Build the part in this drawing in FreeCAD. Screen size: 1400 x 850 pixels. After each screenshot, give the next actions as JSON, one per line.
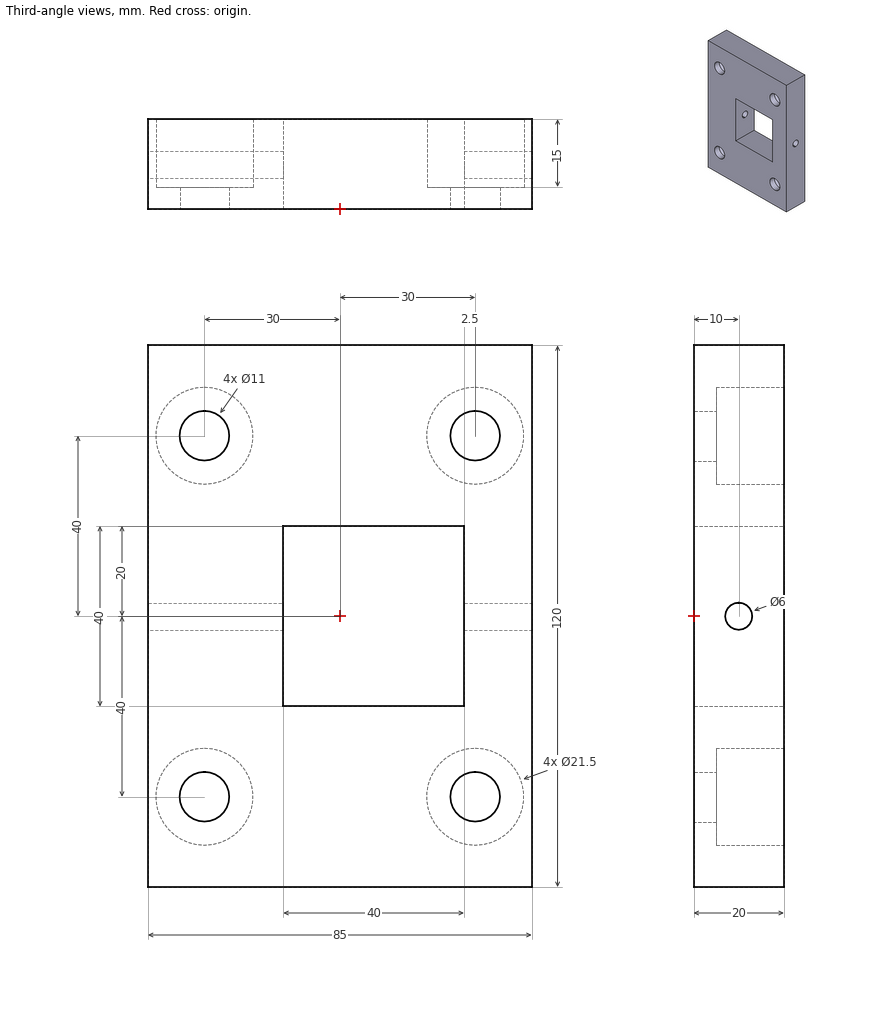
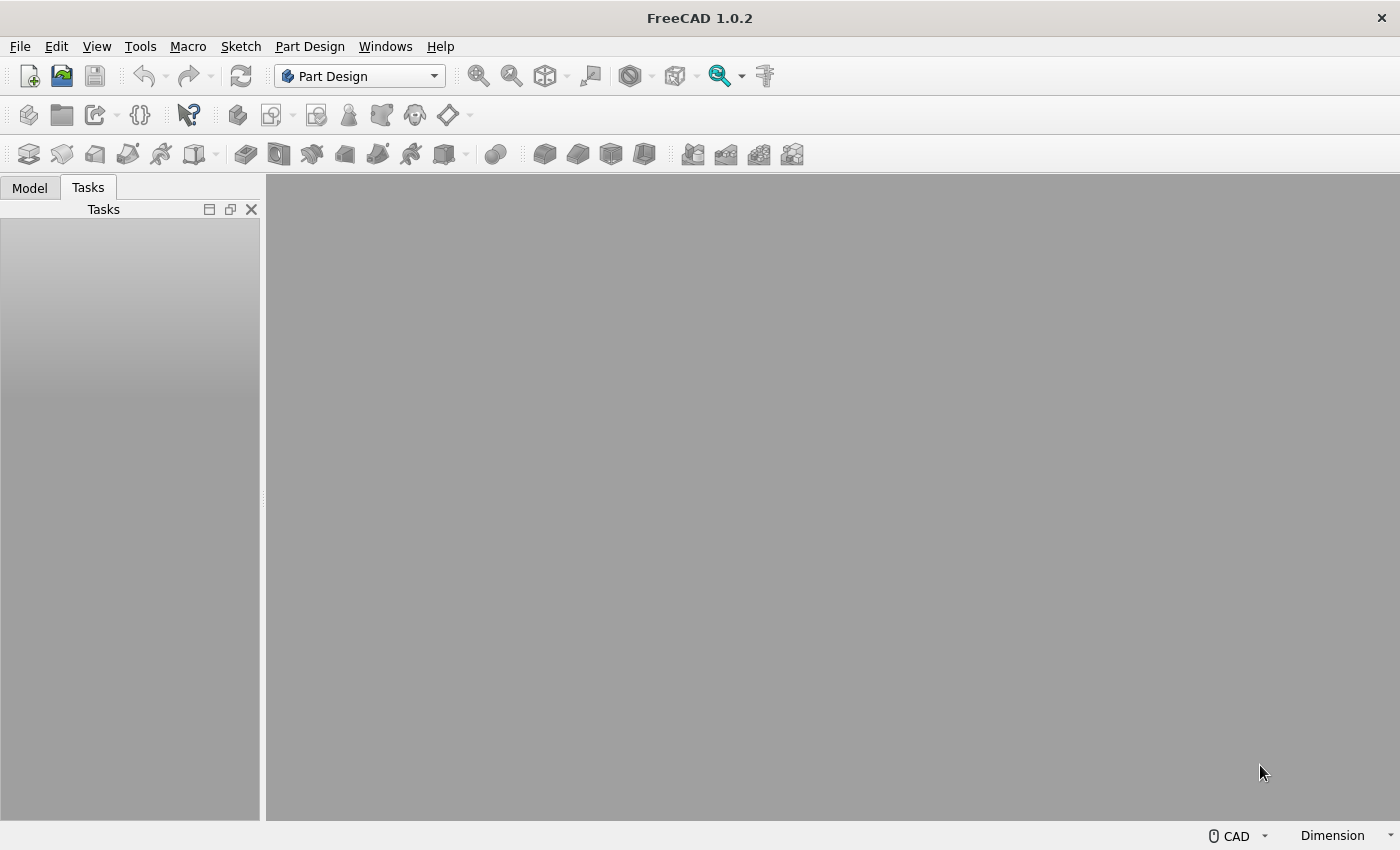
{"action": "key", "text": "ctrl+n"}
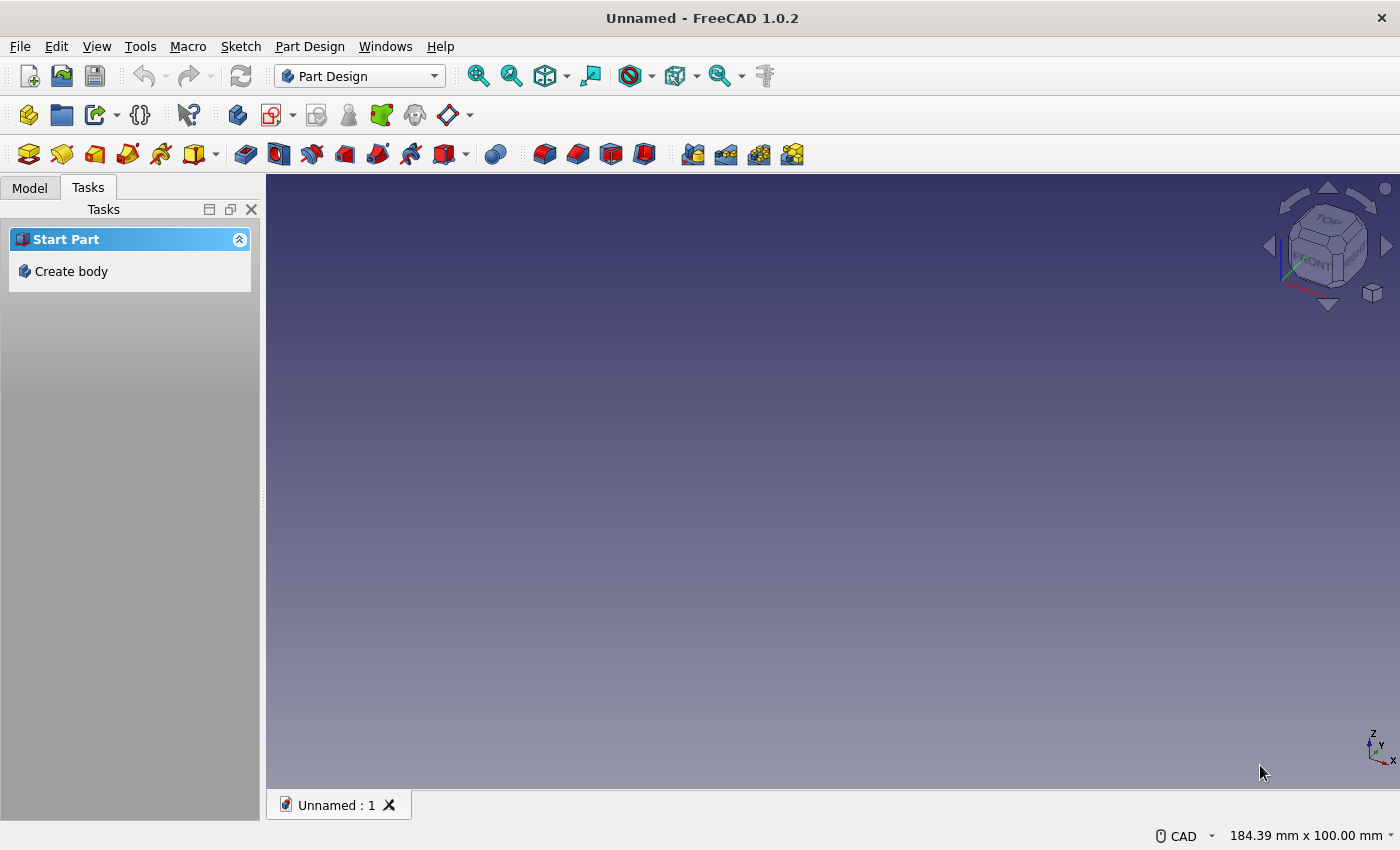
{"action": "left_click", "coordinate": [270, 116]}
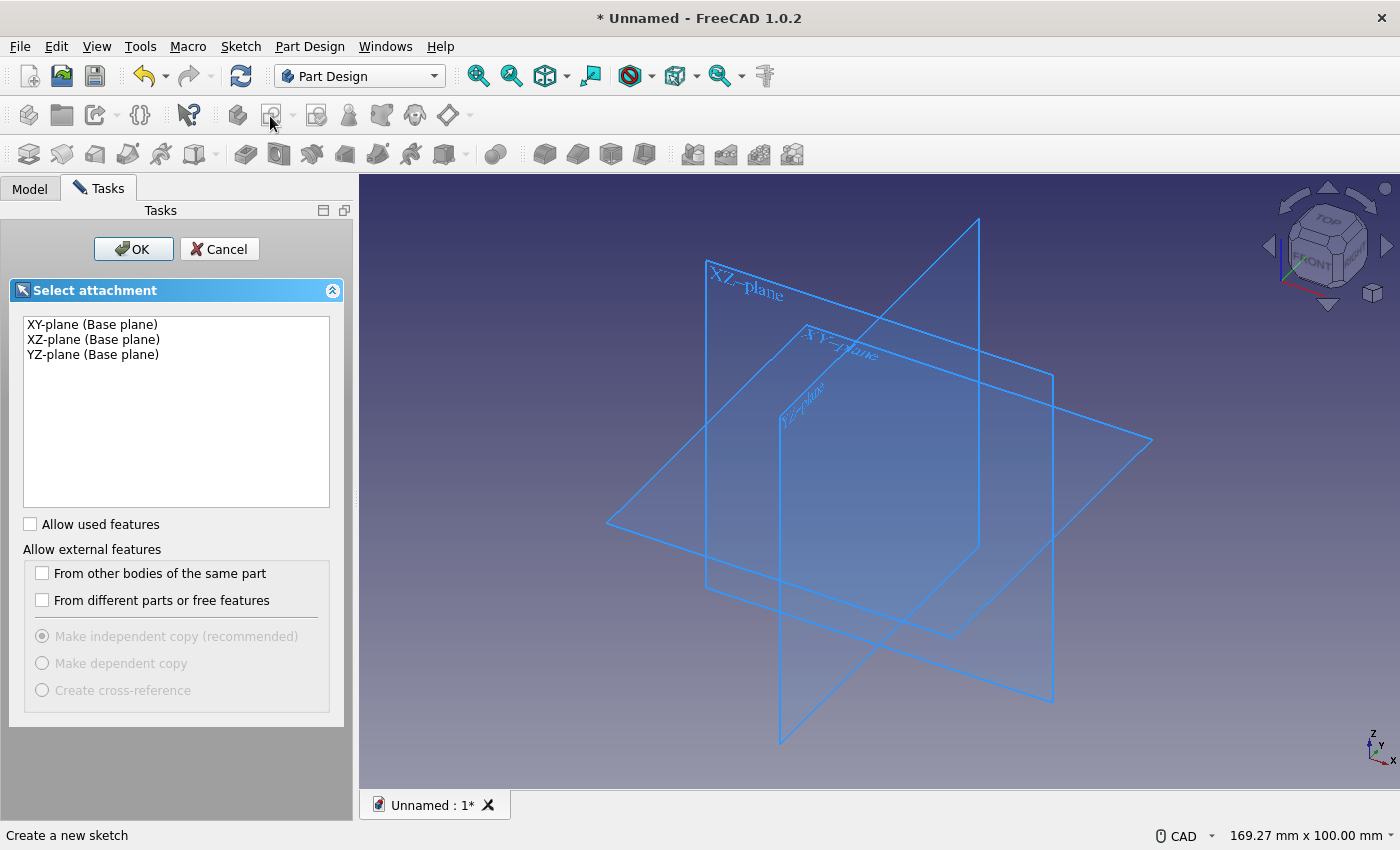
{"action": "left_click", "coordinate": [84, 340]}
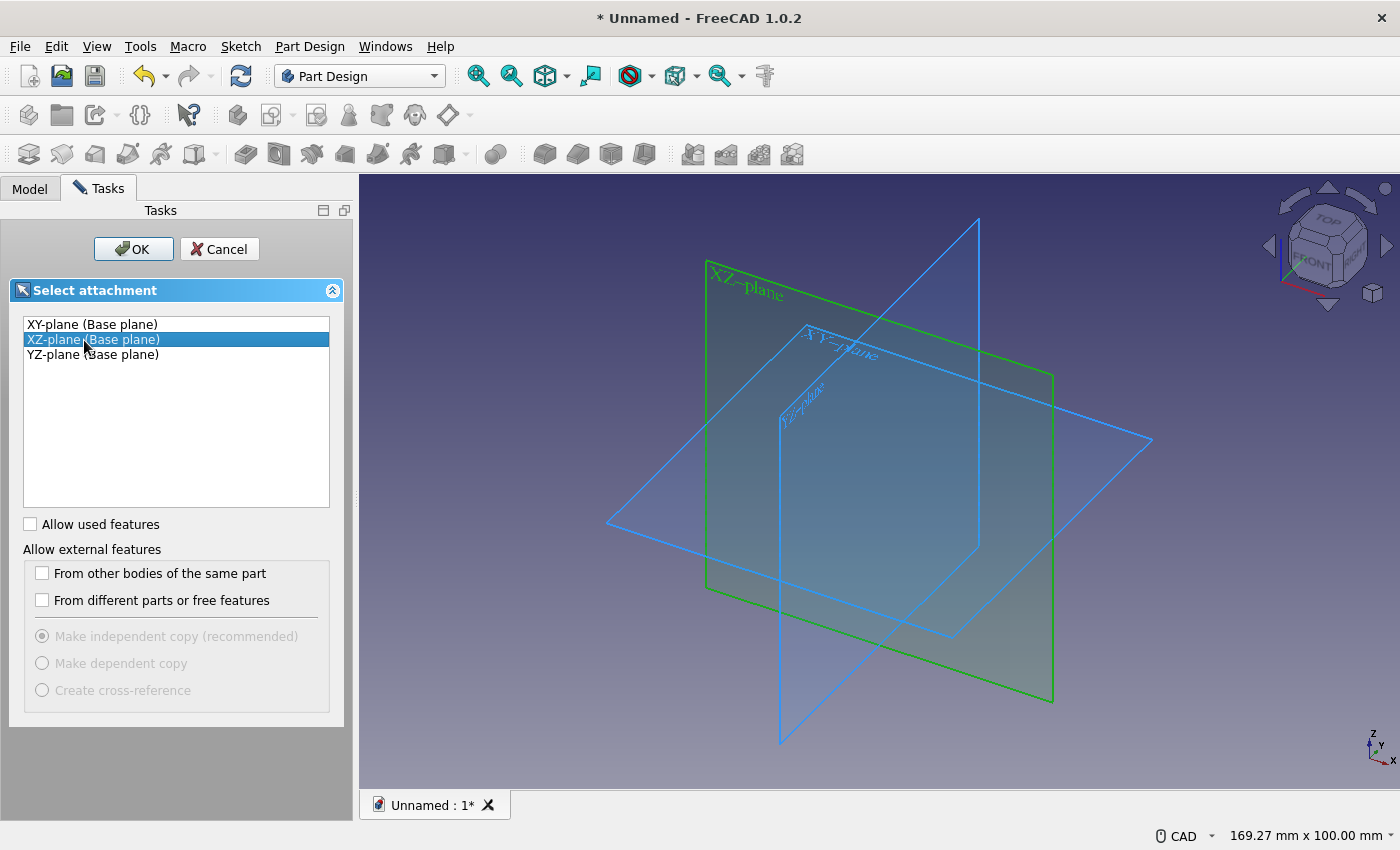
{"action": "left_click", "coordinate": [134, 249]}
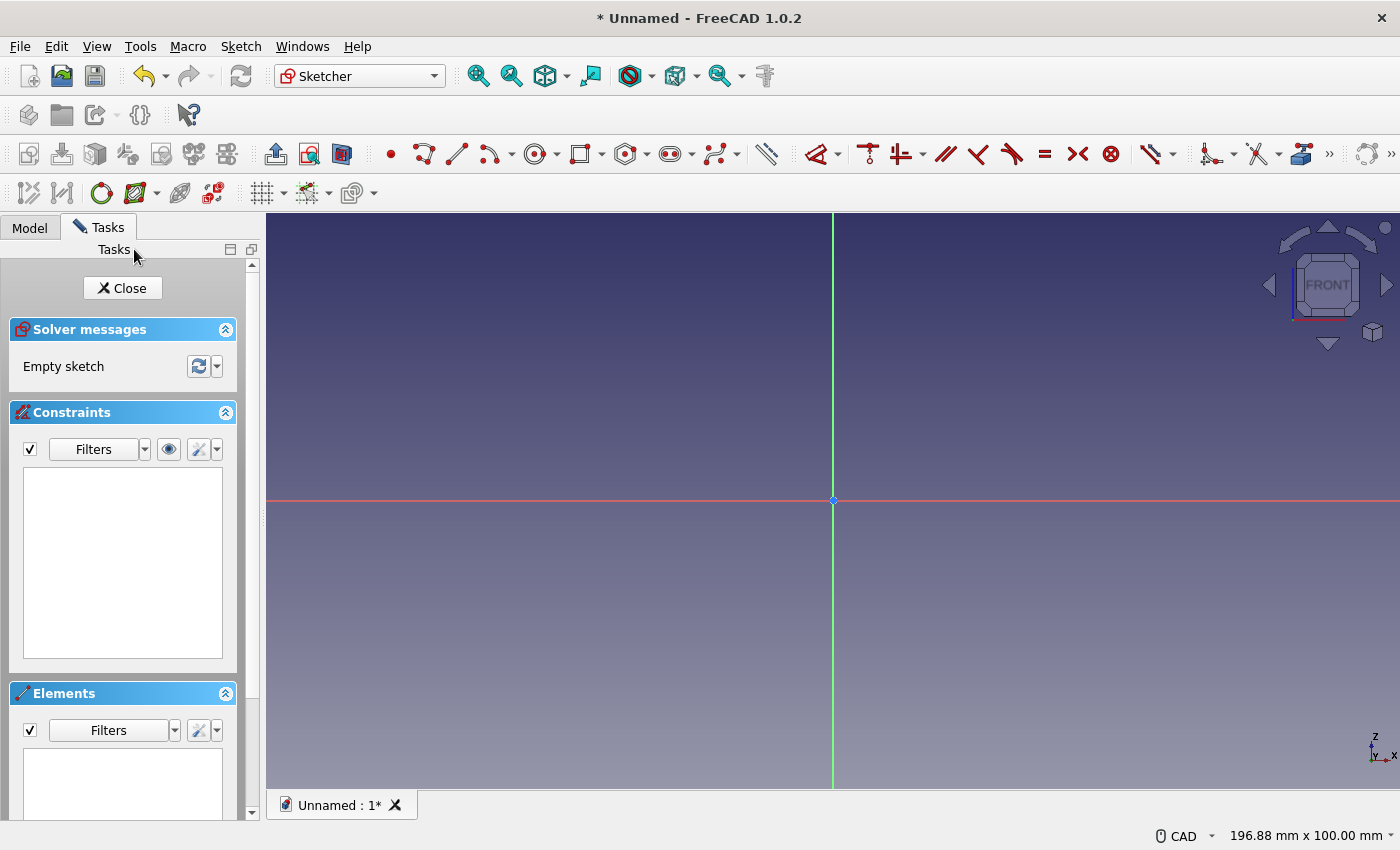
{"action": "scroll", "coordinate": [681, 501], "scroll_direction": "down", "scroll_amount": 3}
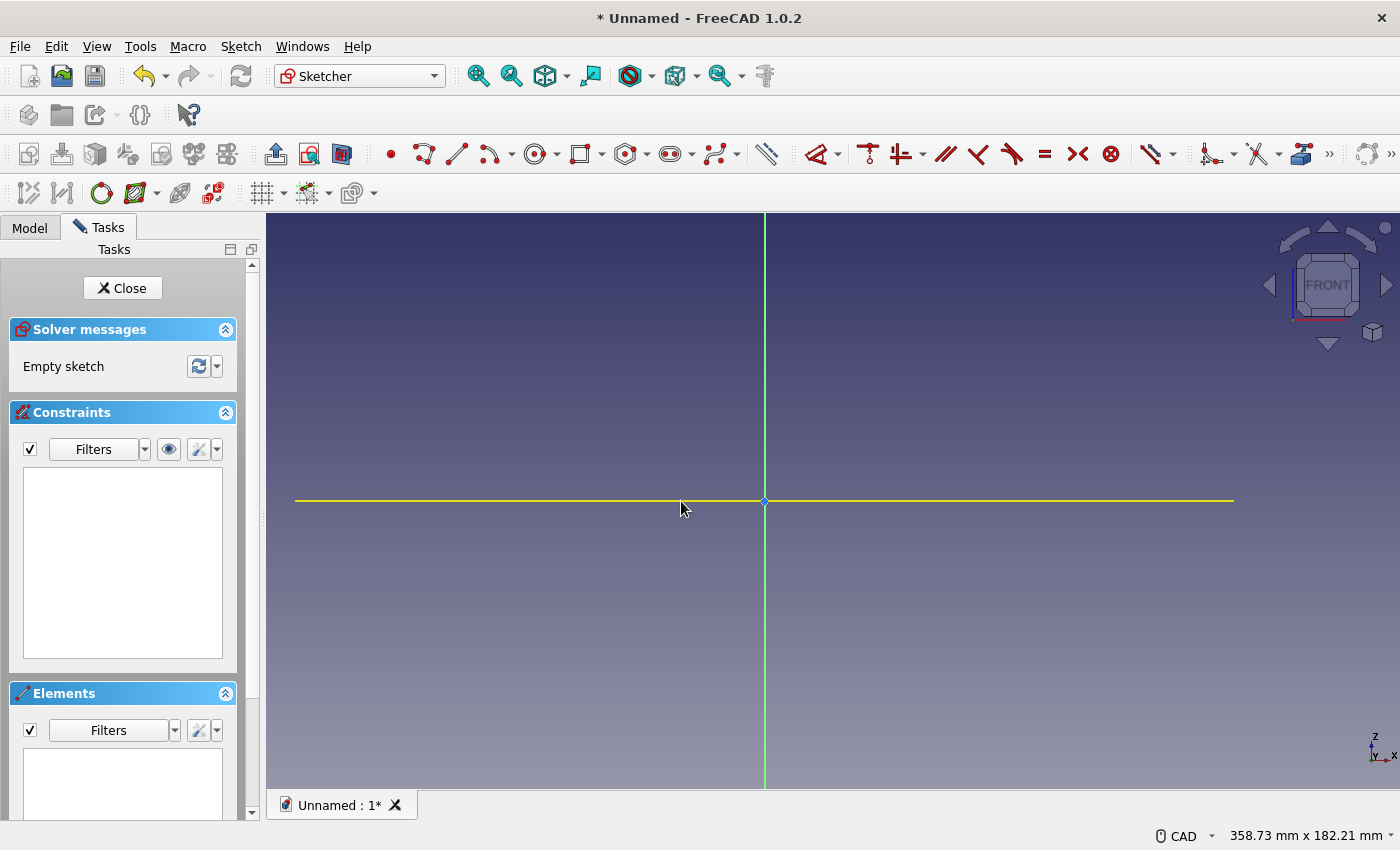
{"action": "left_click", "coordinate": [602, 154]}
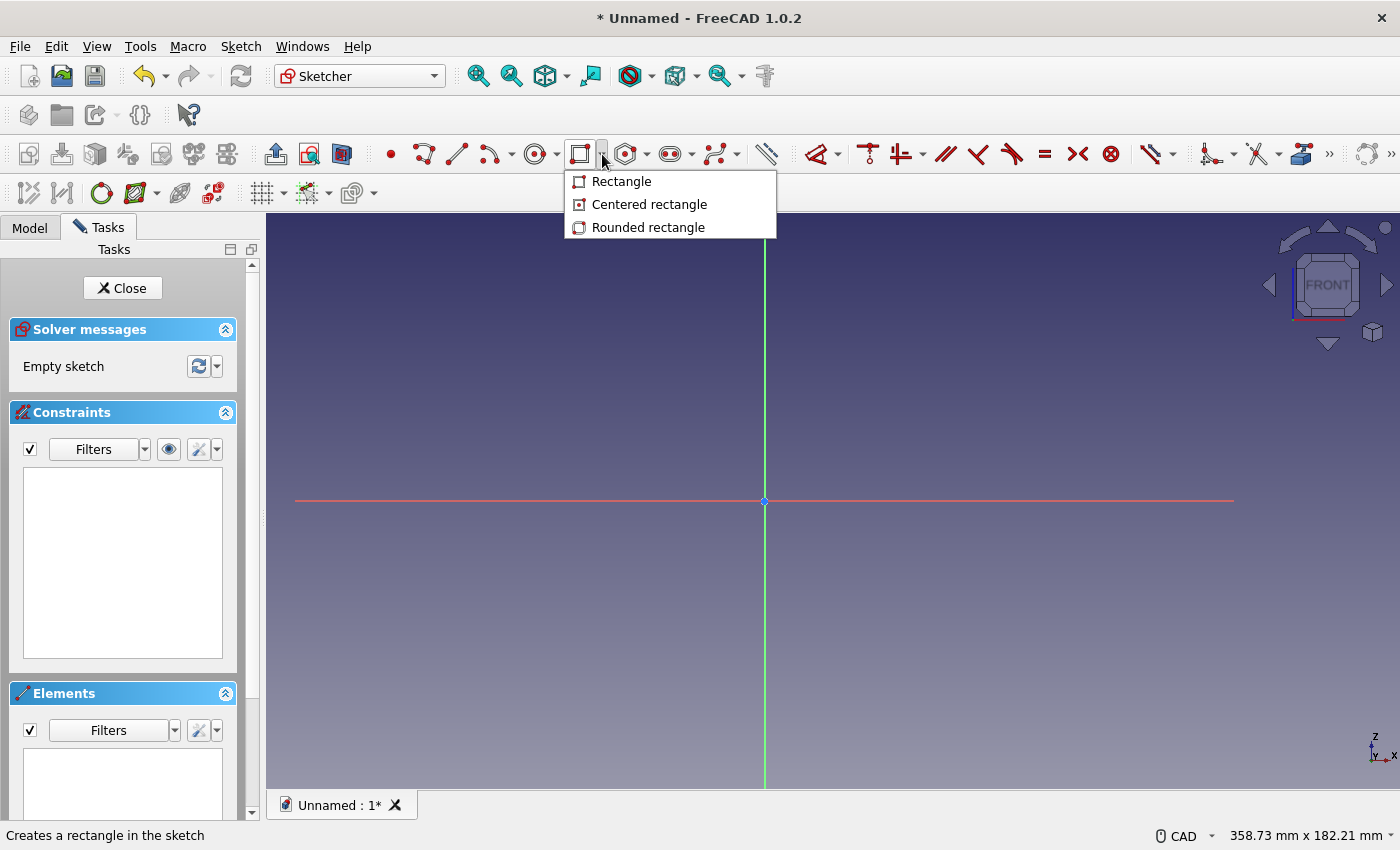
{"action": "left_click", "coordinate": [670, 204]}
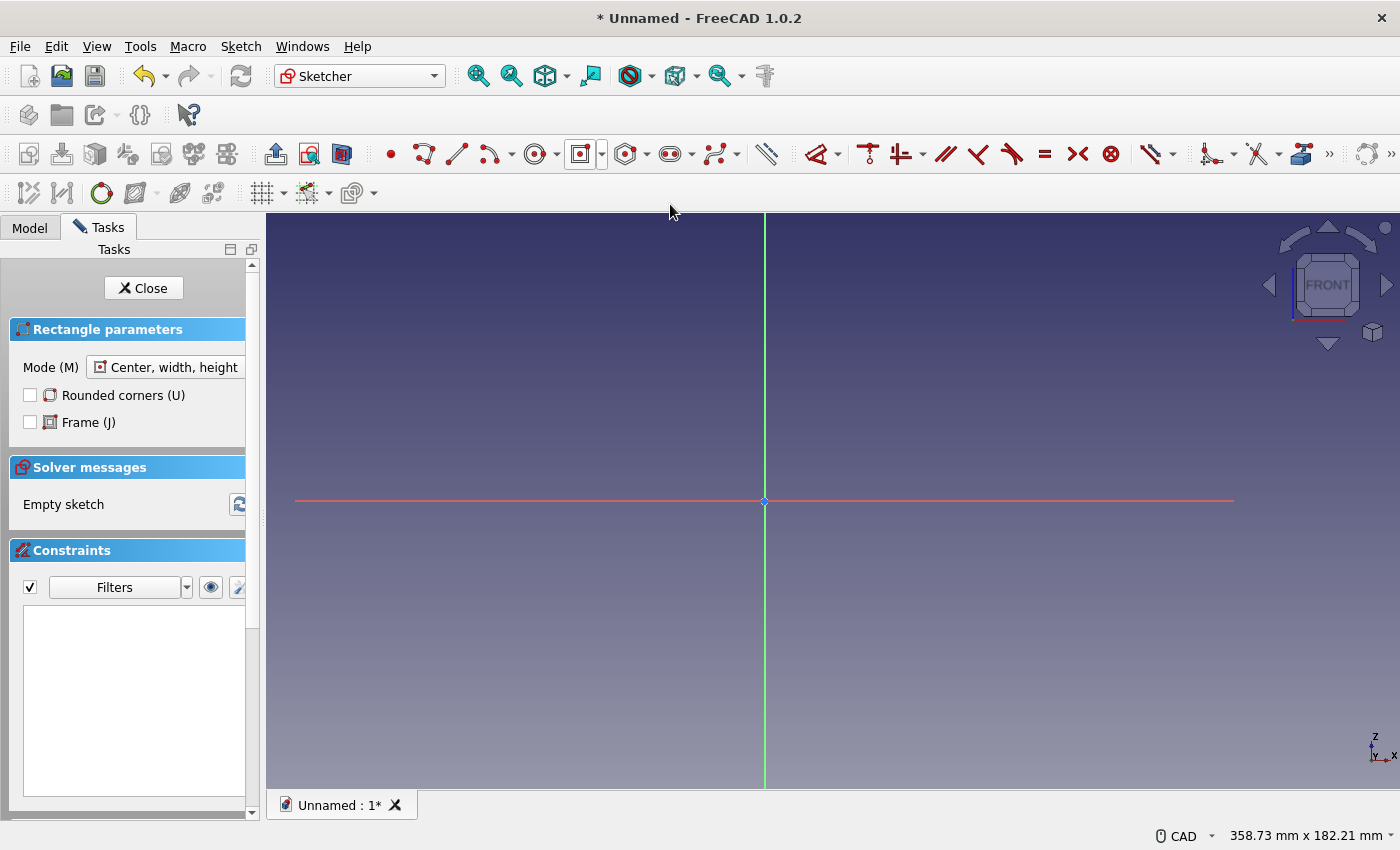
{"action": "left_click", "coordinate": [765, 501]}
{"action": "left_click", "coordinate": [899, 312]}